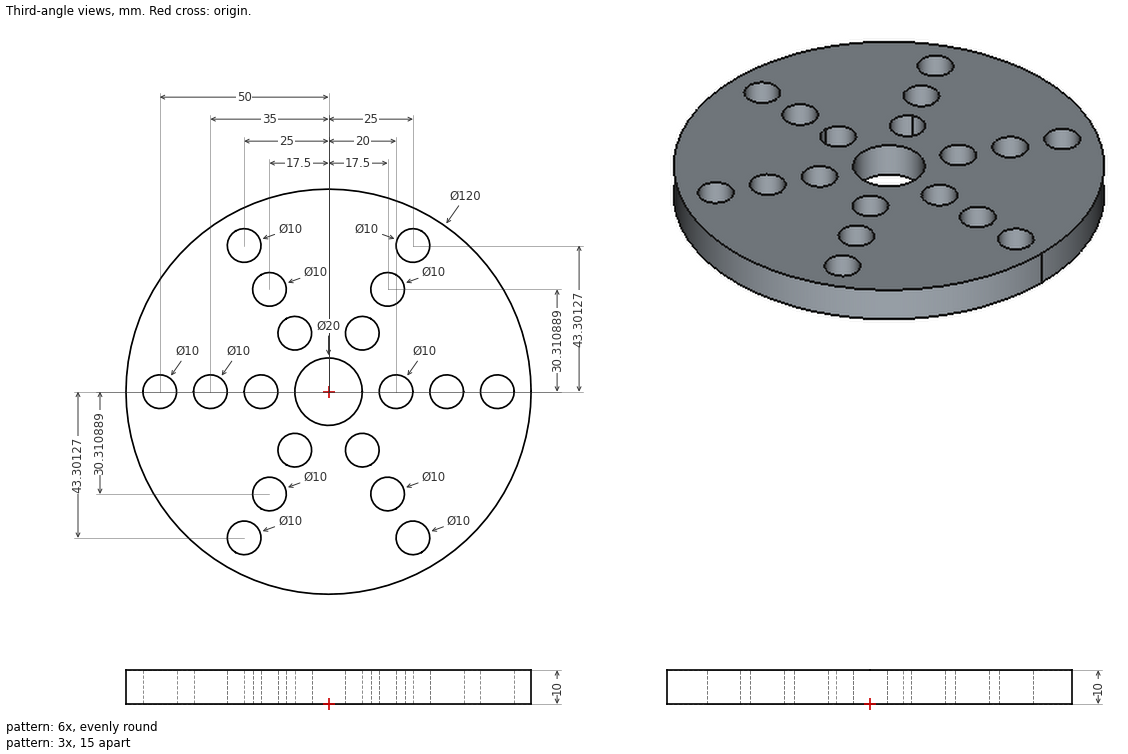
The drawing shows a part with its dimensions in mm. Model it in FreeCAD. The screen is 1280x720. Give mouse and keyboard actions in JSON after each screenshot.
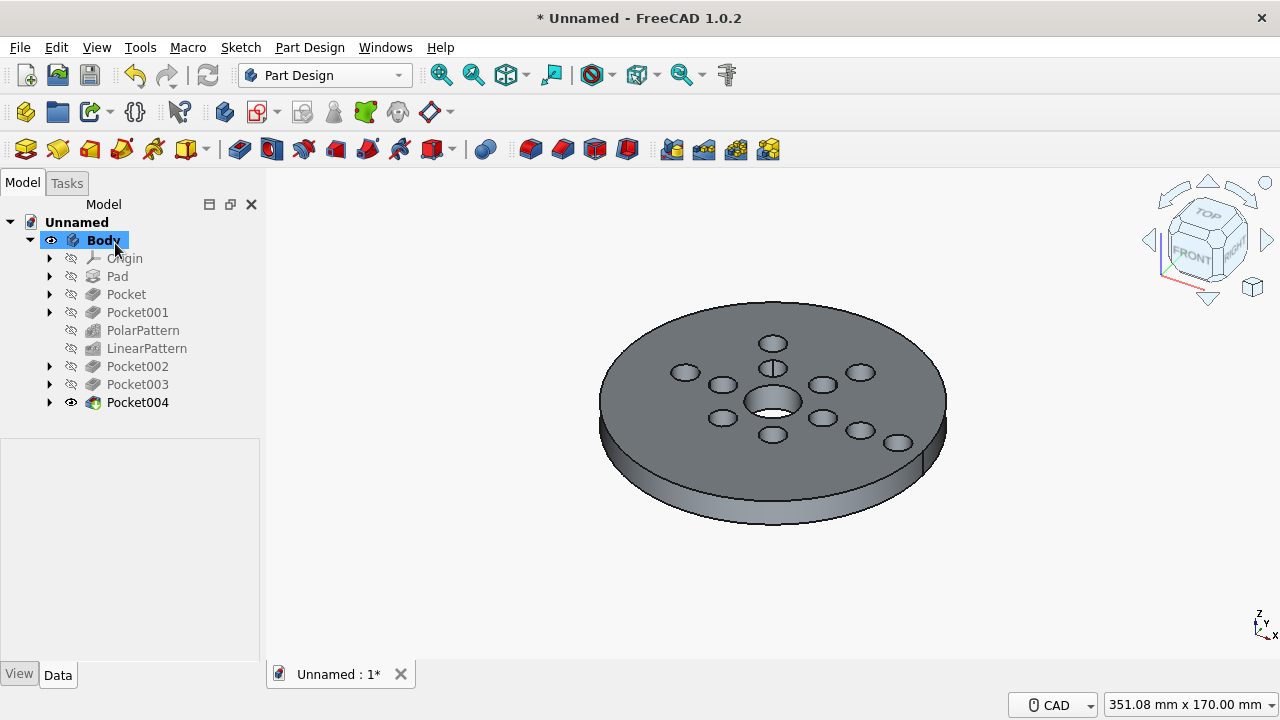
{"action": "left_click", "coordinate": [723, 450]}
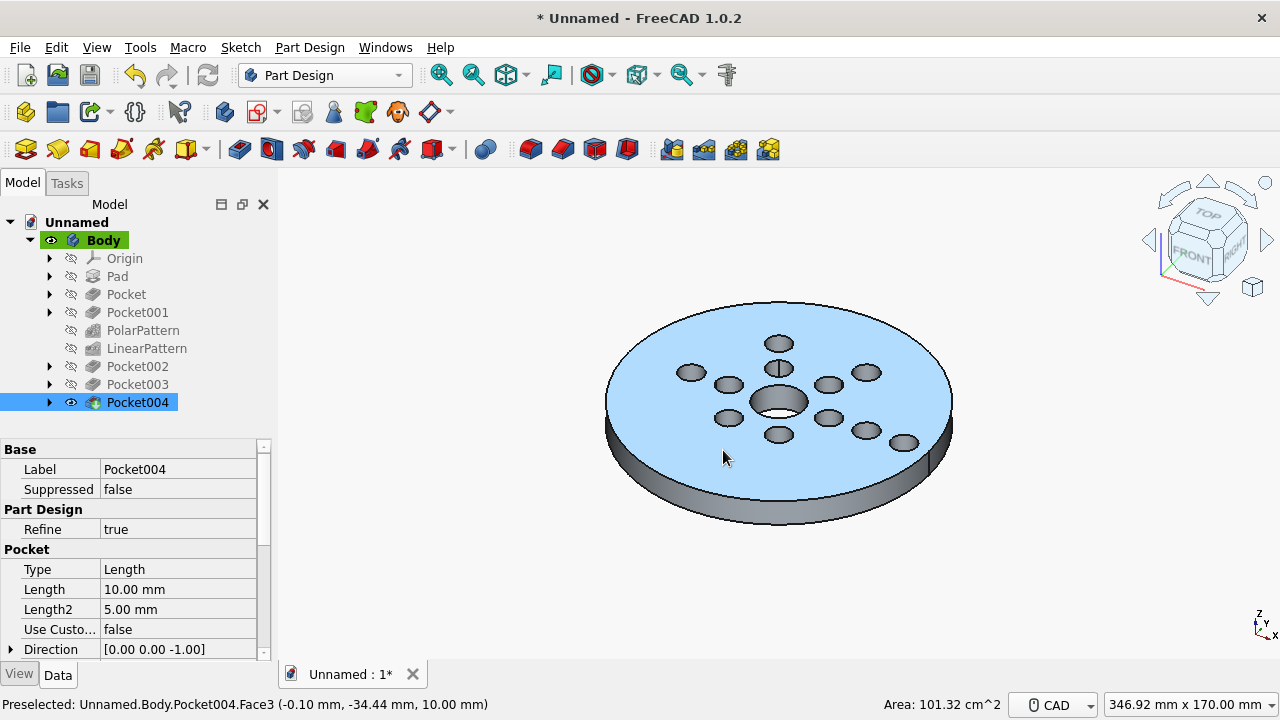
{"action": "left_click", "coordinate": [258, 112]}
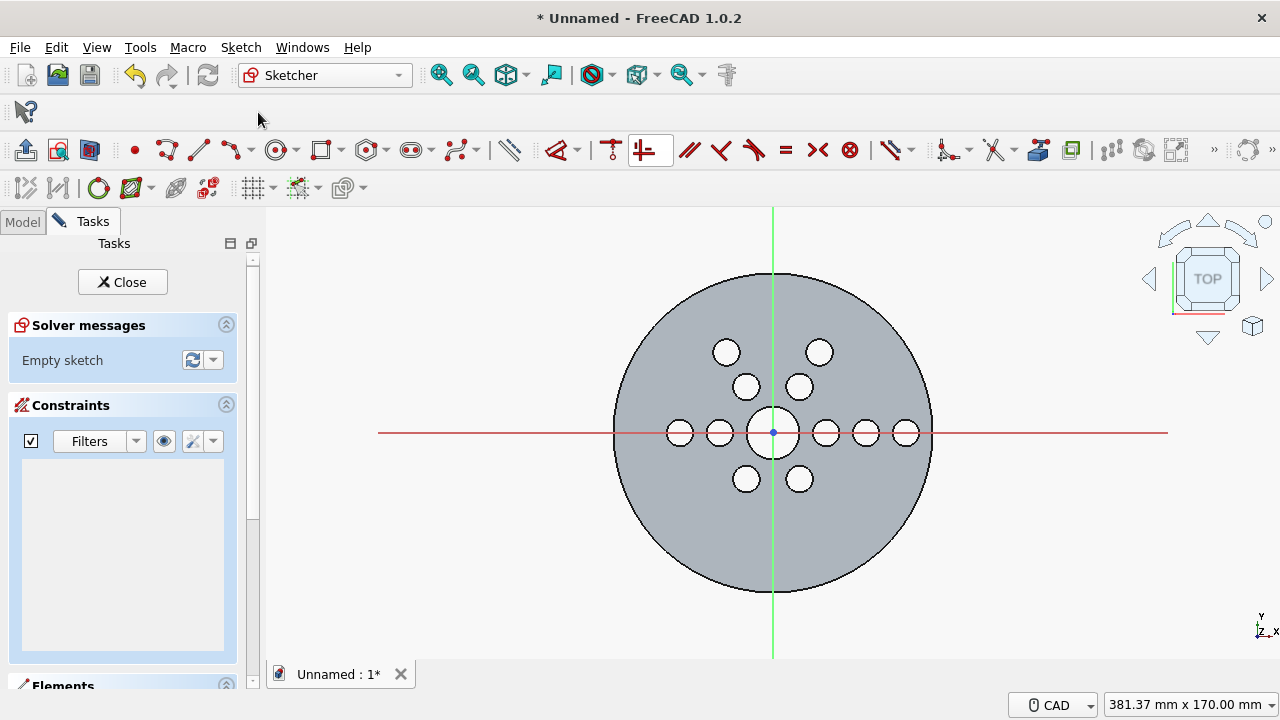
{"action": "scroll", "coordinate": [729, 522], "scroll_direction": "up", "scroll_amount": 12}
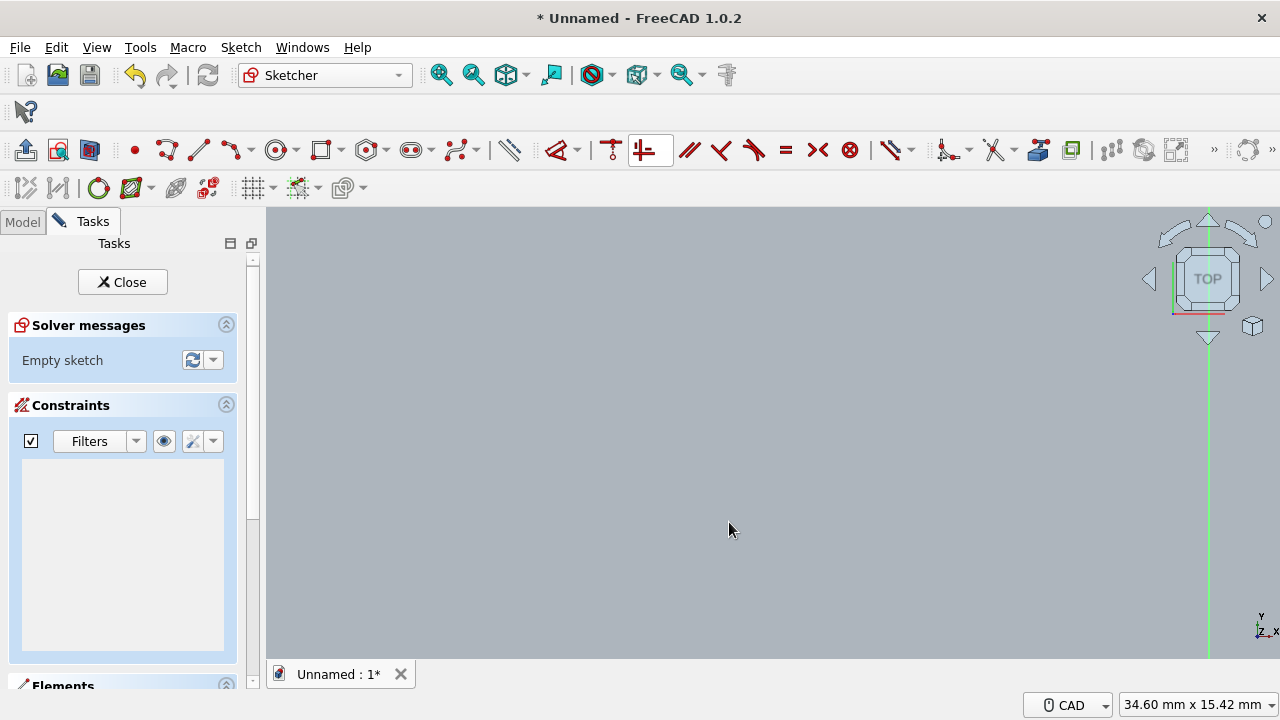
{"action": "left_click", "coordinate": [276, 150]}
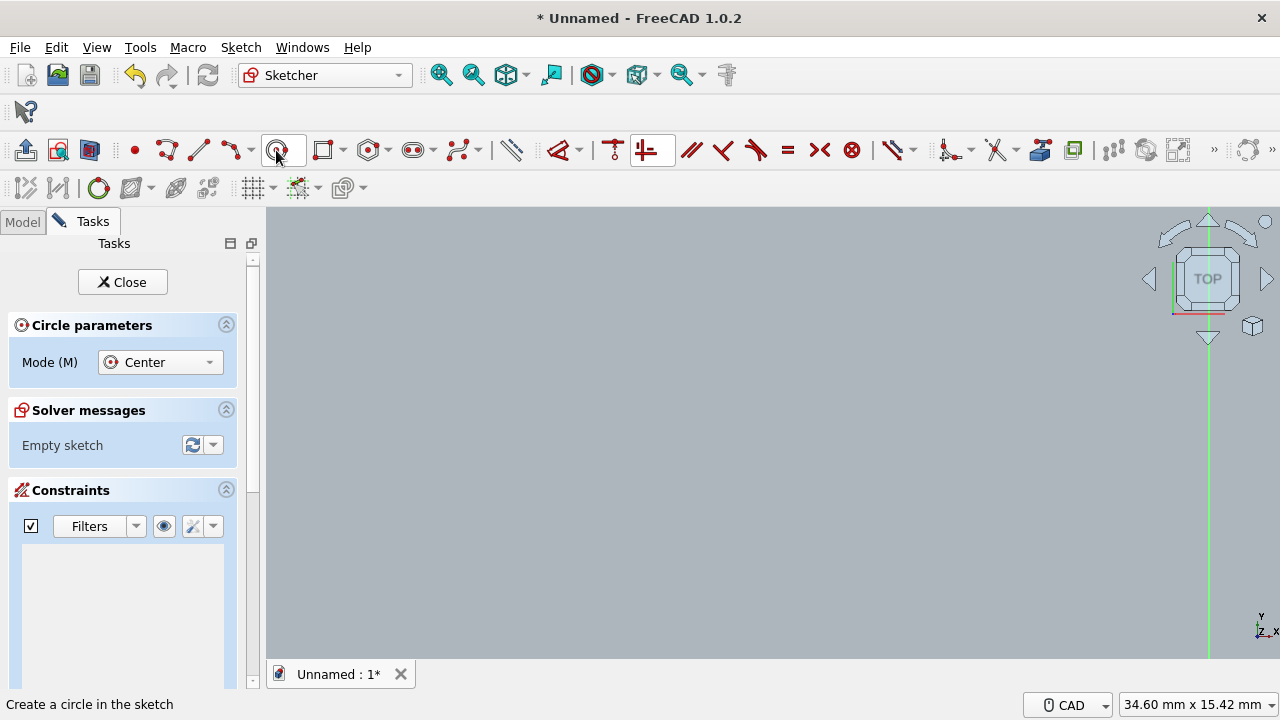
{"action": "left_click", "coordinate": [697, 422]}
{"action": "left_click", "coordinate": [800, 319]}
{"action": "key", "text": "Escape"}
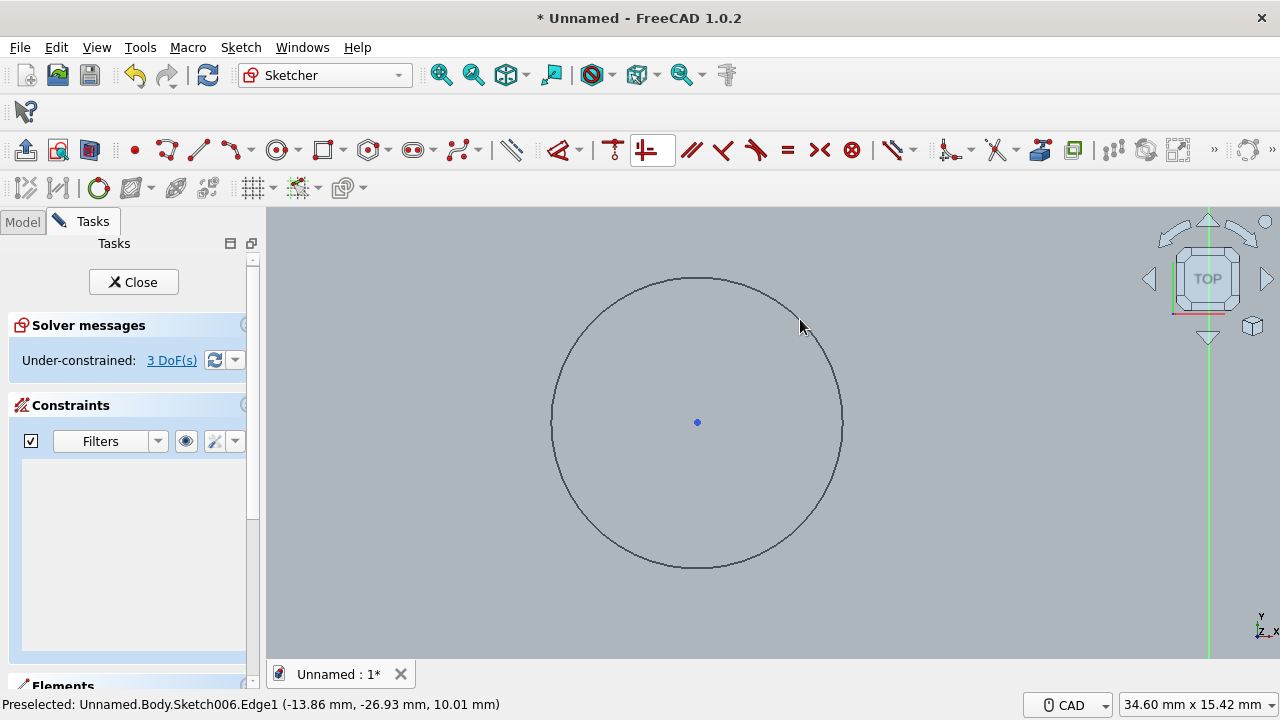
{"action": "left_click", "coordinate": [558, 150]}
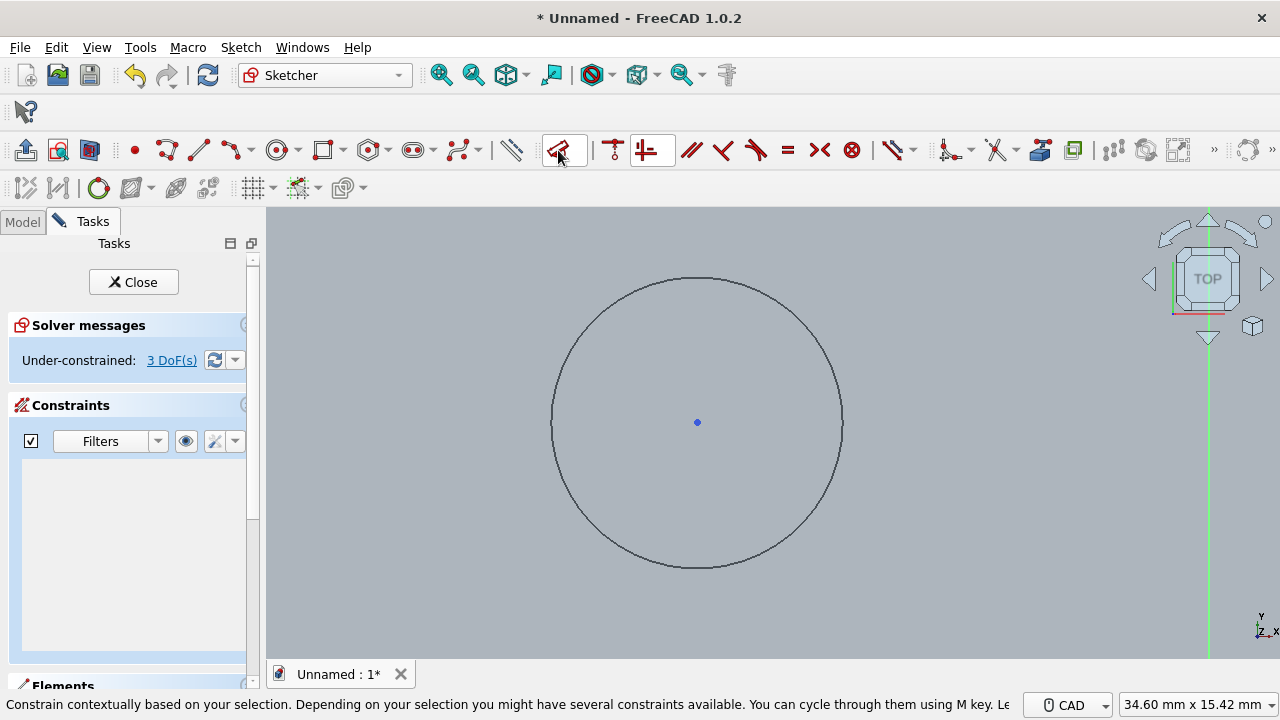
{"action": "left_click", "coordinate": [800, 320]}
{"action": "left_click", "coordinate": [823, 297]}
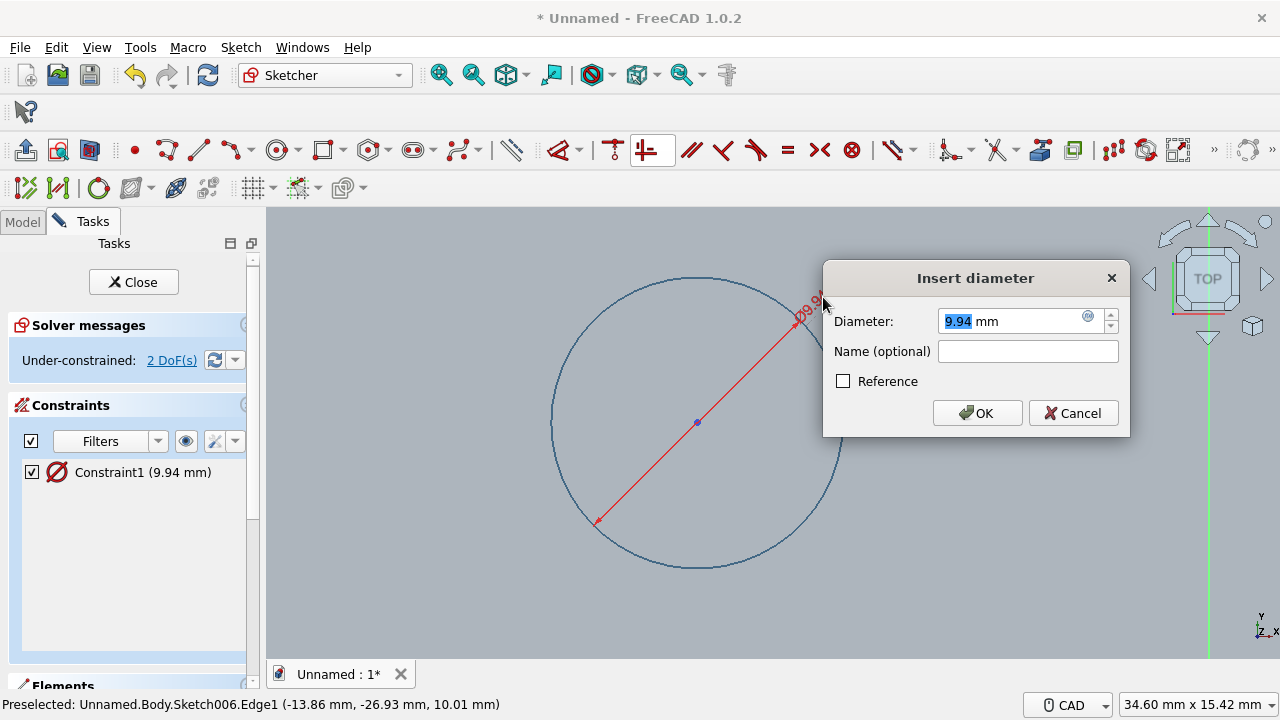
{"action": "type", "text": "10"}
{"action": "key", "text": "Return"}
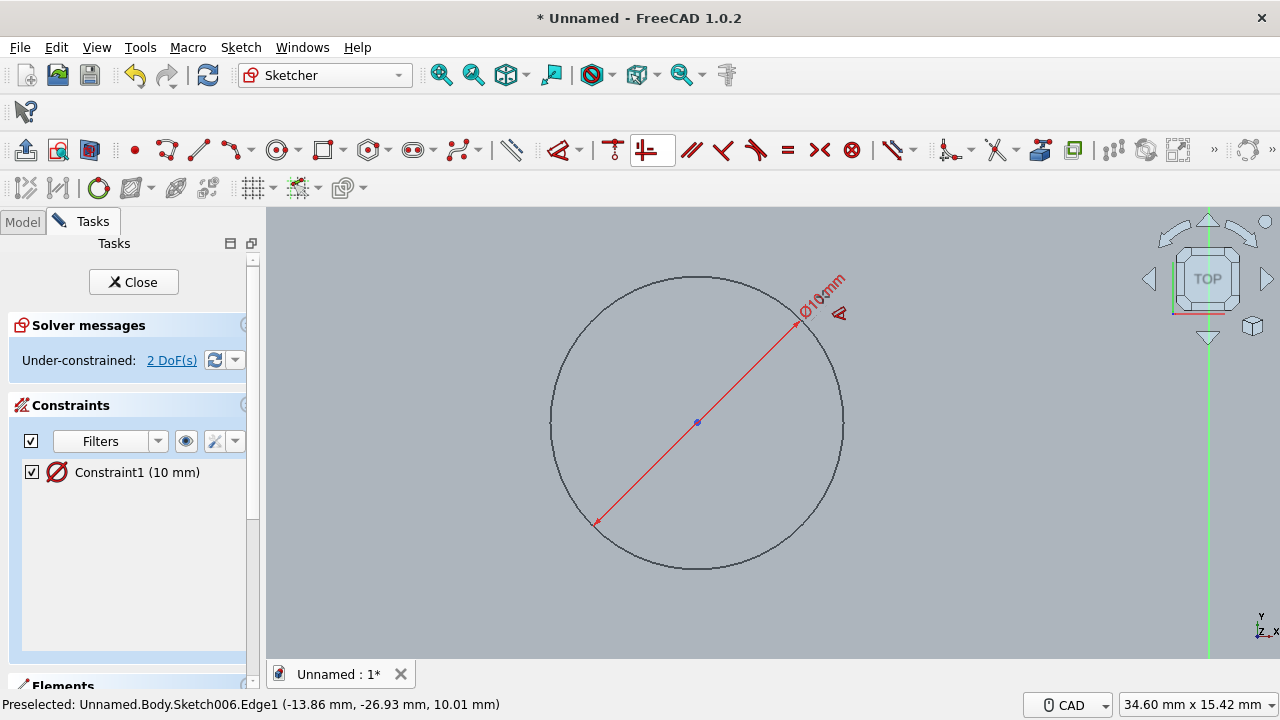
{"action": "left_click", "coordinate": [697, 423]}
{"action": "left_click", "coordinate": [906, 457]}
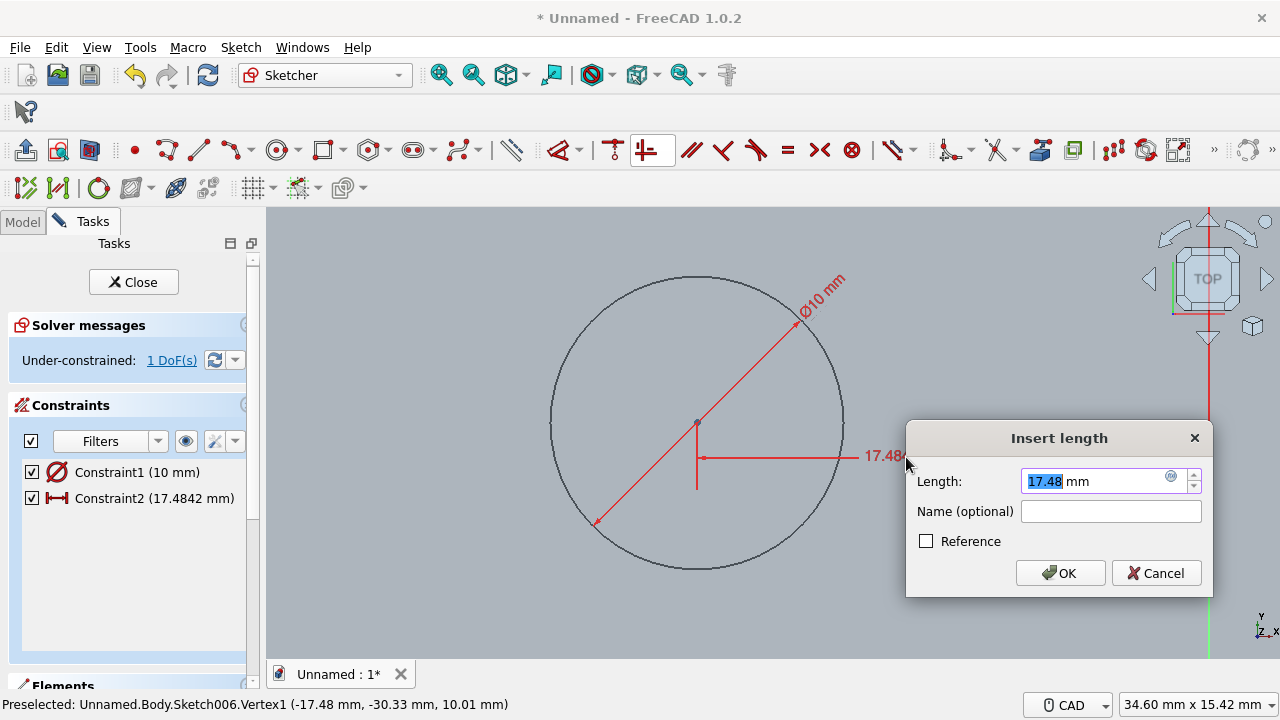
{"action": "type", "text": "17.5"}
{"action": "key", "text": "Return"}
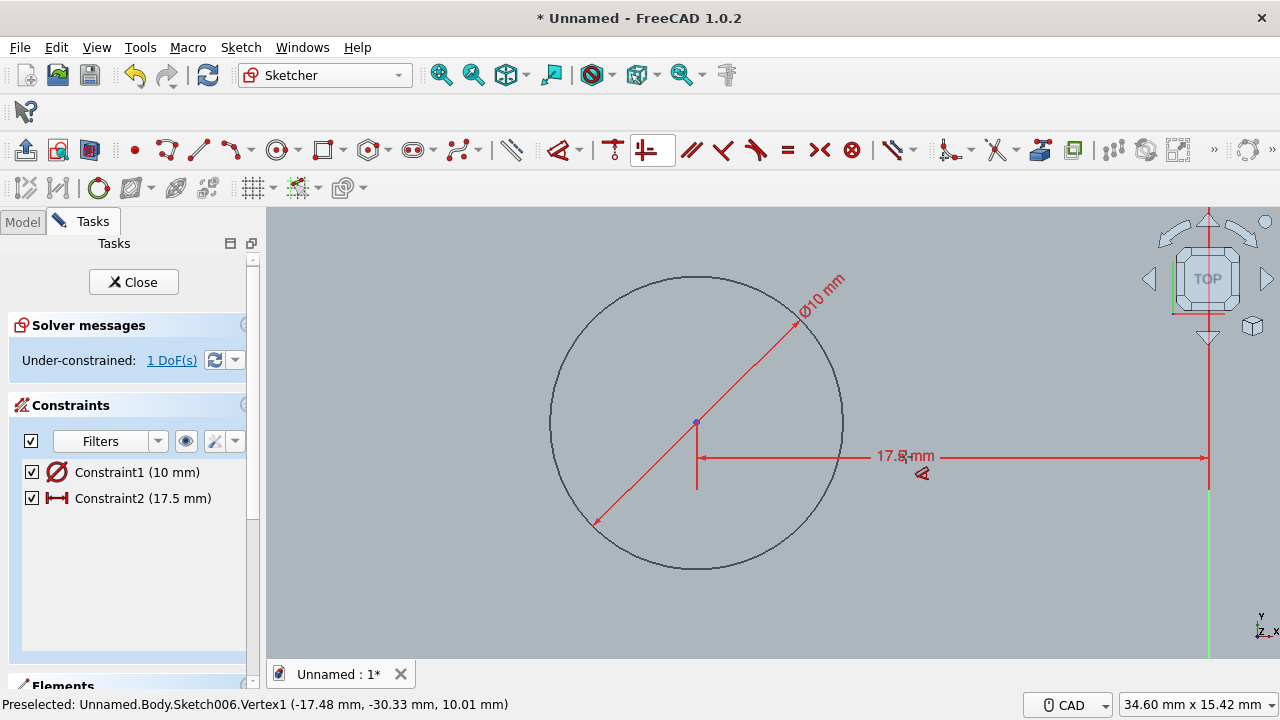
{"action": "left_click", "coordinate": [697, 423]}
{"action": "left_click", "coordinate": [663, 329]}